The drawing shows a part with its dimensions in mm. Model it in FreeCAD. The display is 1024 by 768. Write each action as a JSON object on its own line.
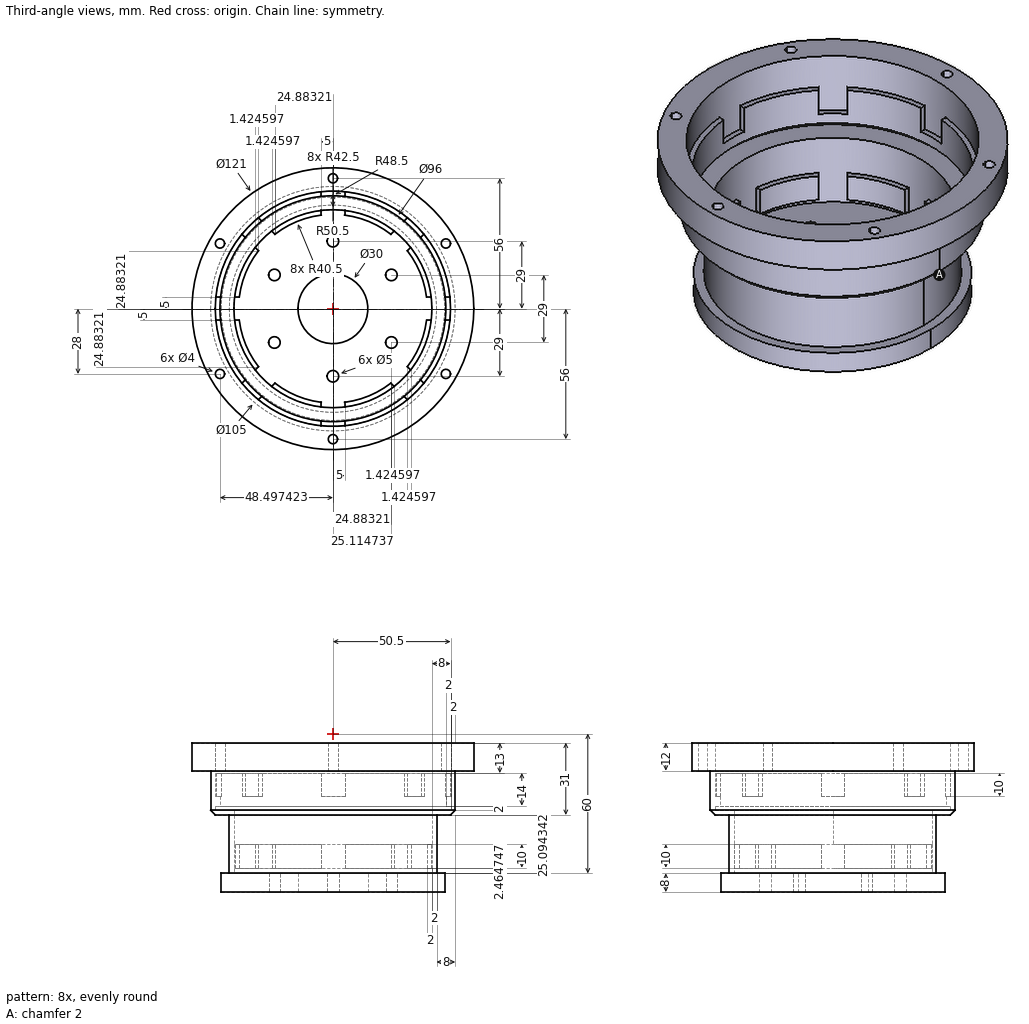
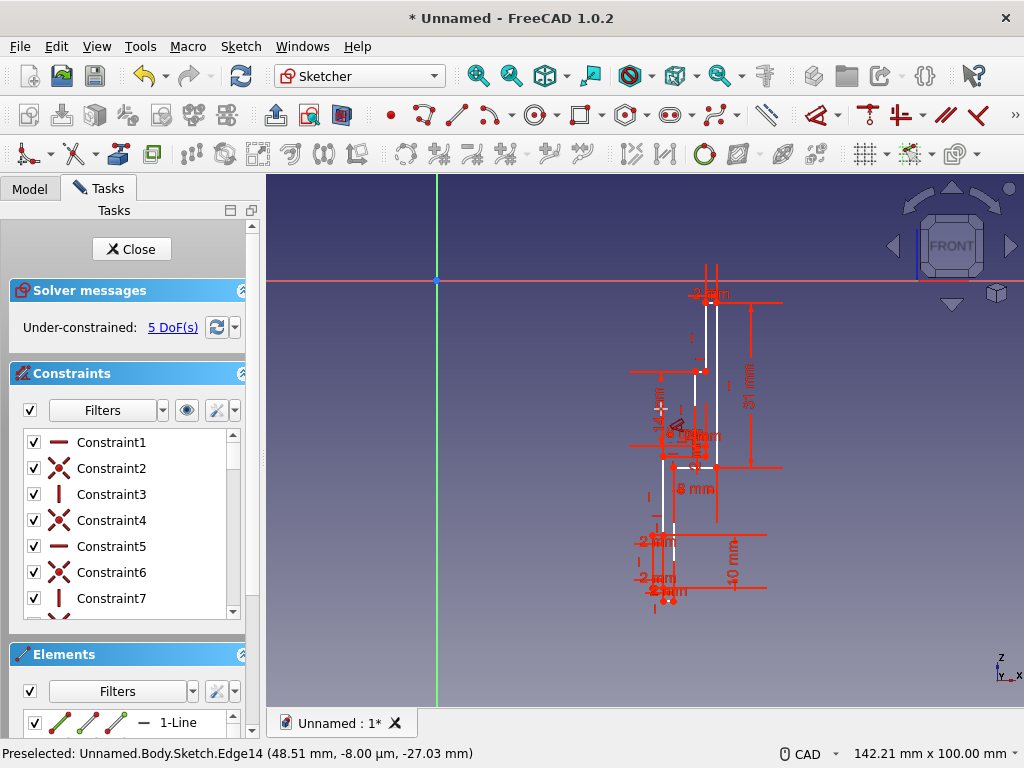
{"action": "scroll", "coordinate": [706, 351], "scroll_direction": "up", "scroll_amount": 2}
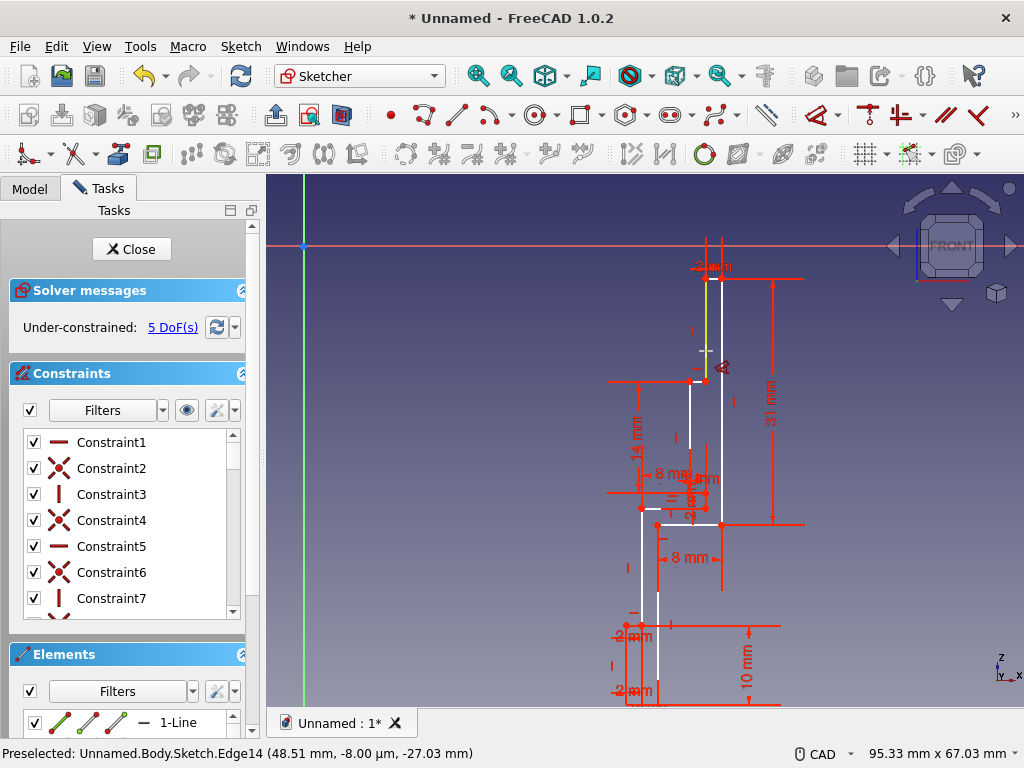
{"action": "left_click", "coordinate": [706, 351]}
{"action": "left_click", "coordinate": [740, 330]}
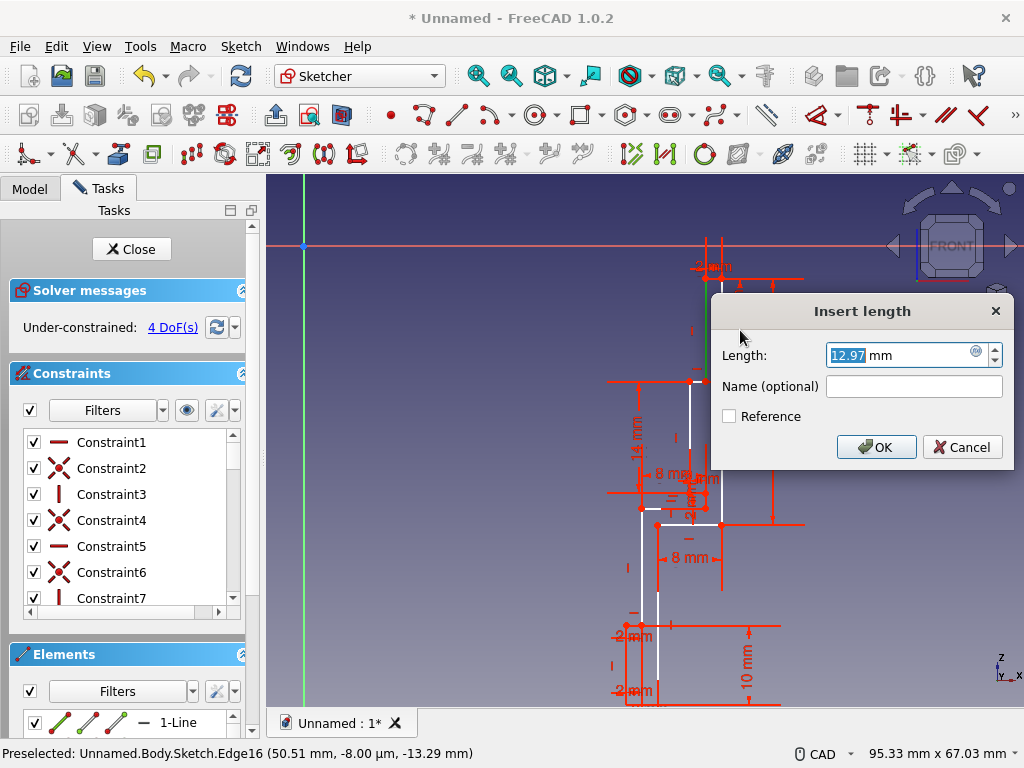
{"action": "type", "text": "13"}
{"action": "key", "text": "Return"}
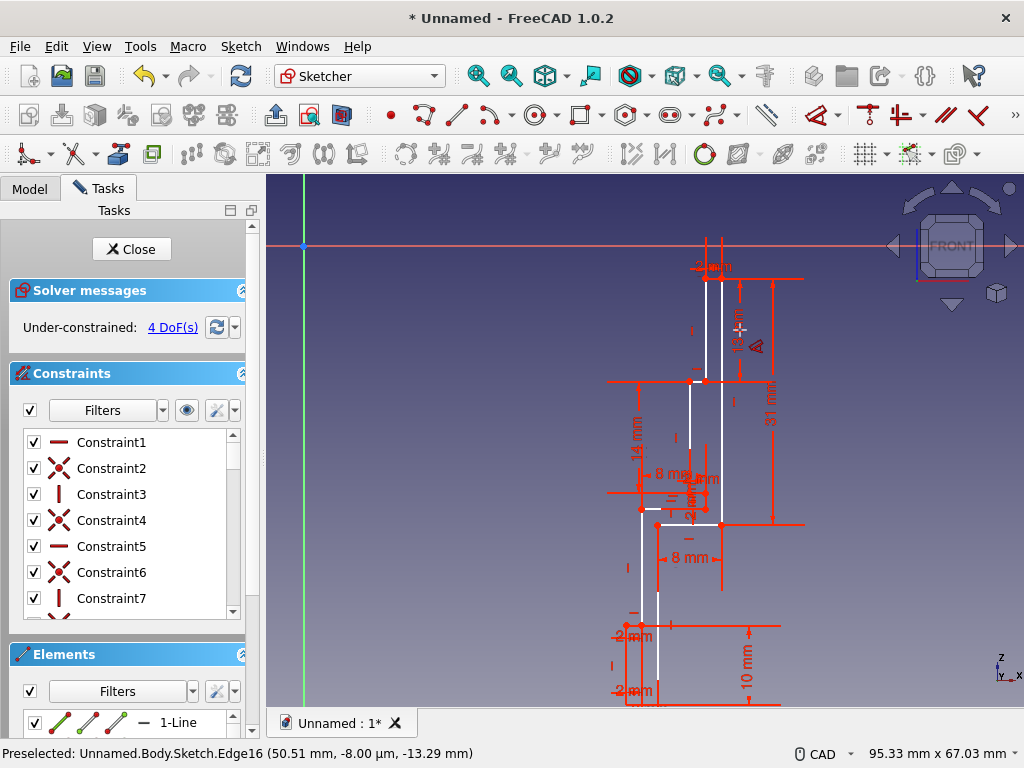
{"action": "scroll", "coordinate": [706, 350], "scroll_direction": "down", "scroll_amount": 2}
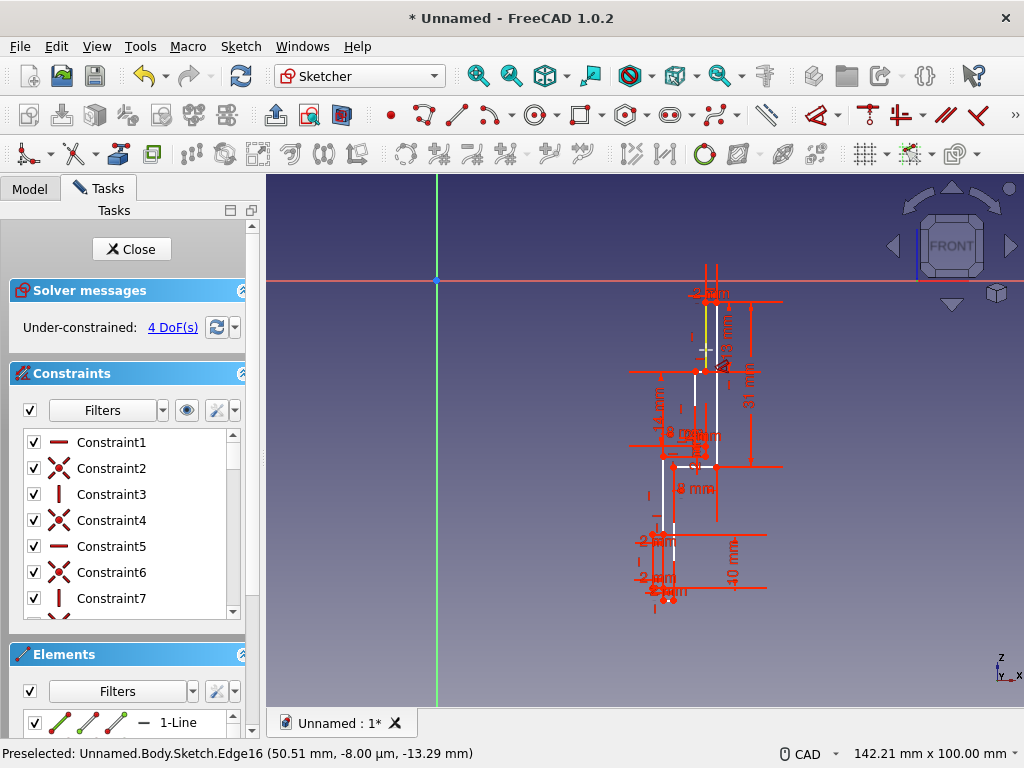
{"action": "left_click", "coordinate": [674, 601]}
{"action": "left_click", "coordinate": [403, 441]}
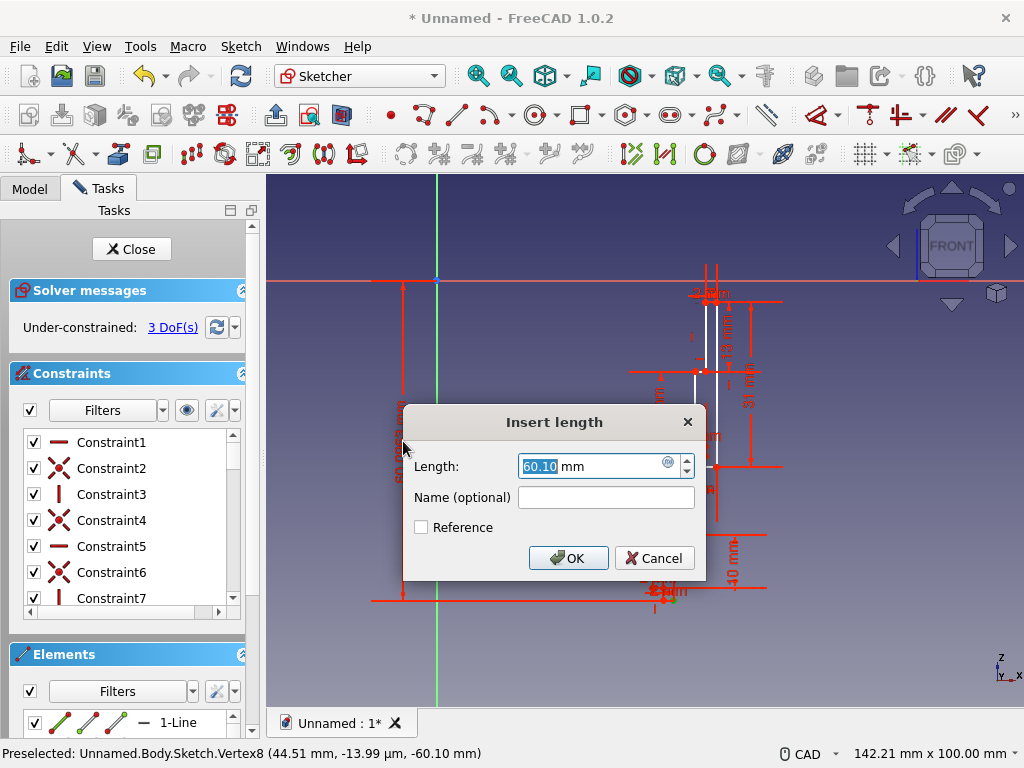
{"action": "type", "text": "60"}
{"action": "key", "text": "Return"}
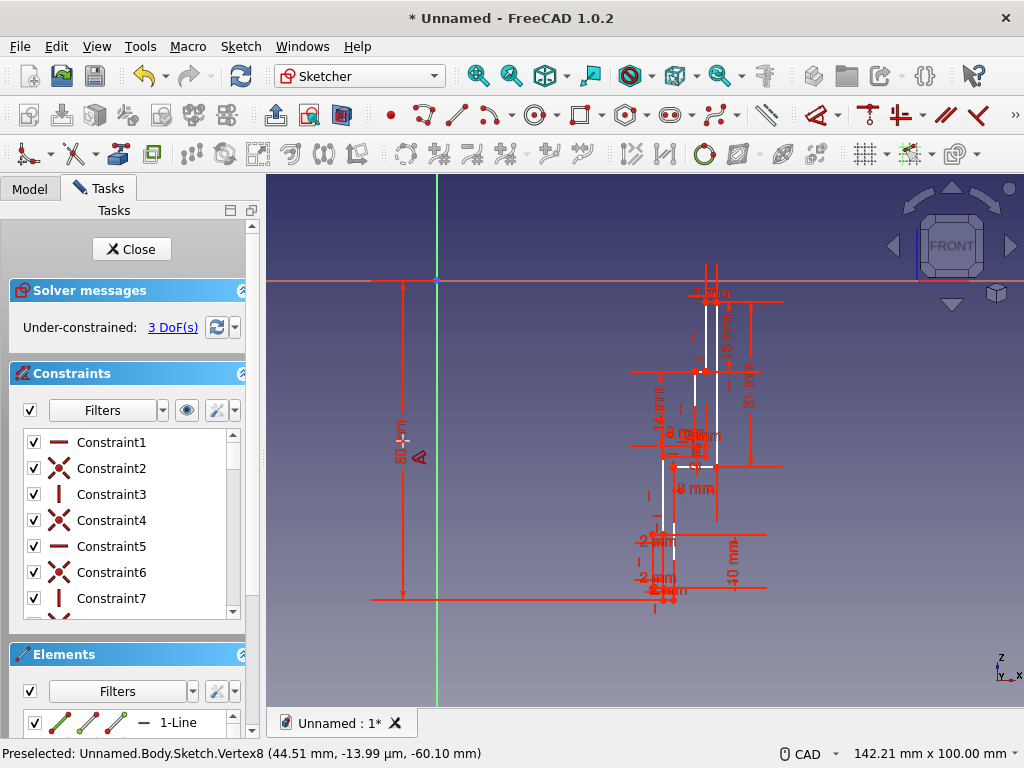
{"action": "left_click", "coordinate": [706, 302]}
{"action": "left_click", "coordinate": [571, 247]}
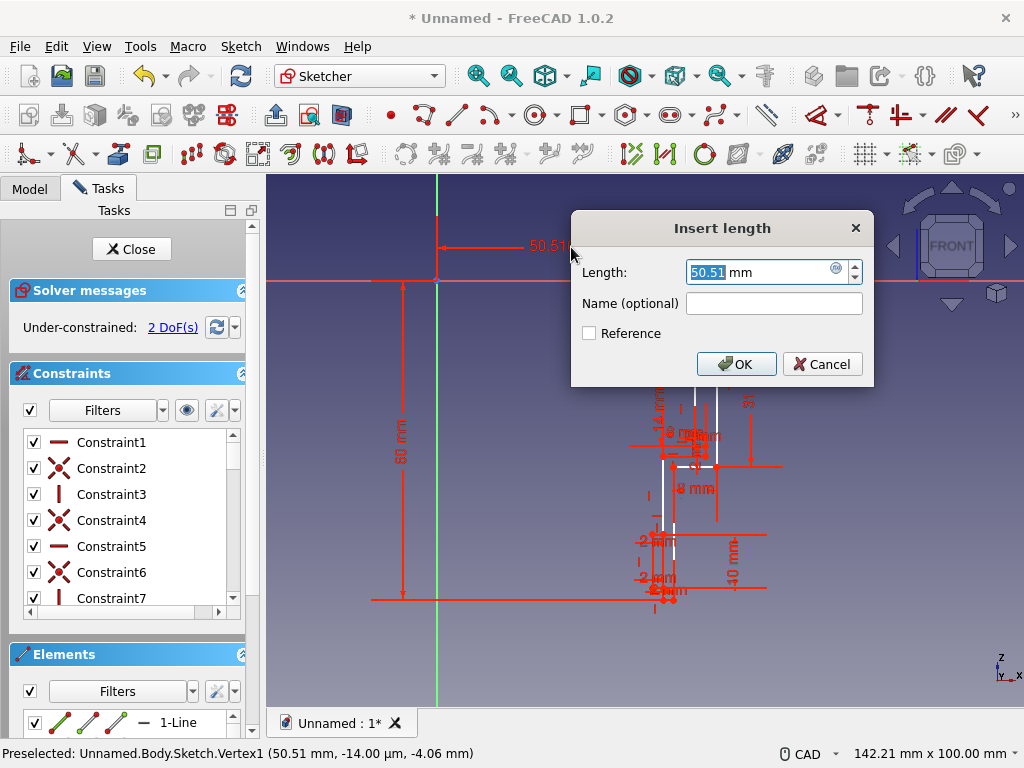
{"action": "type", "text": "50.5"}
{"action": "key", "text": "Return"}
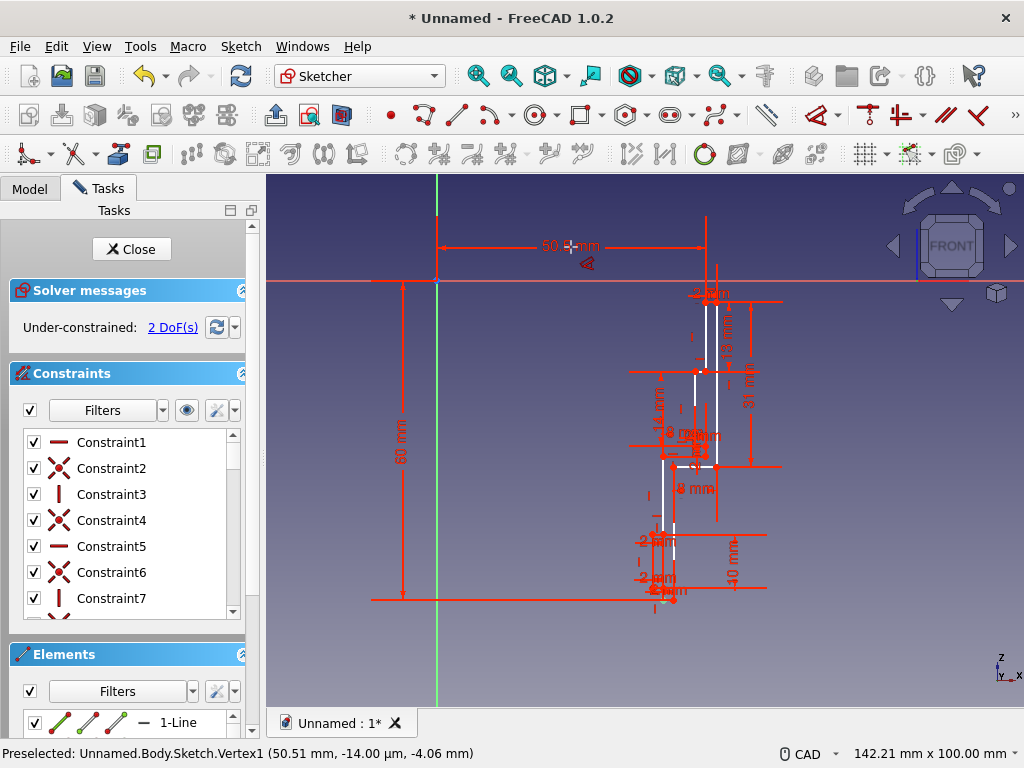
{"action": "scroll", "coordinate": [663, 594], "scroll_direction": "up", "scroll_amount": 6}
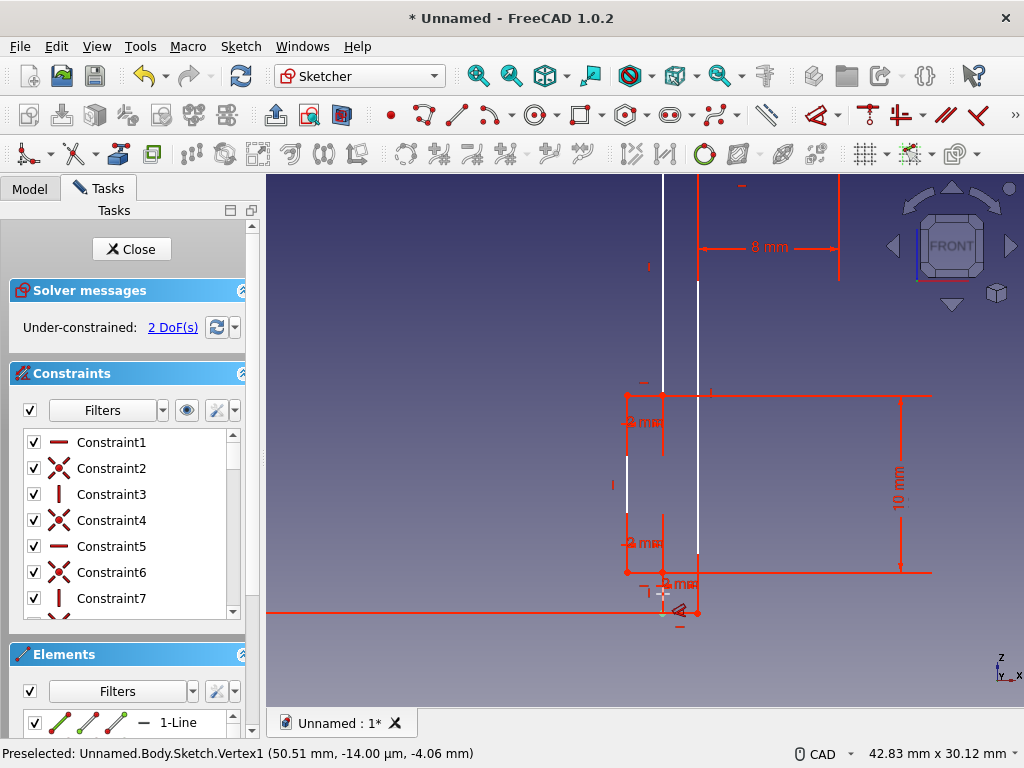
{"action": "left_click", "coordinate": [663, 593]}
{"action": "left_click", "coordinate": [629, 607]}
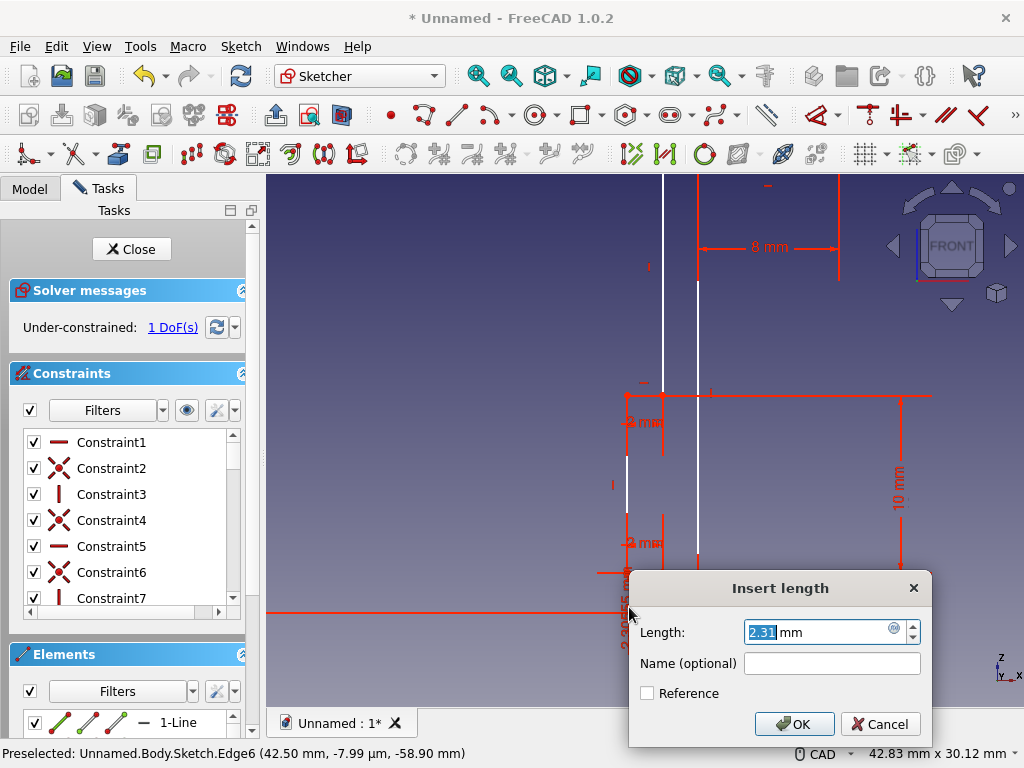
{"action": "type", "text": "2.464747"}
{"action": "key", "text": "Return"}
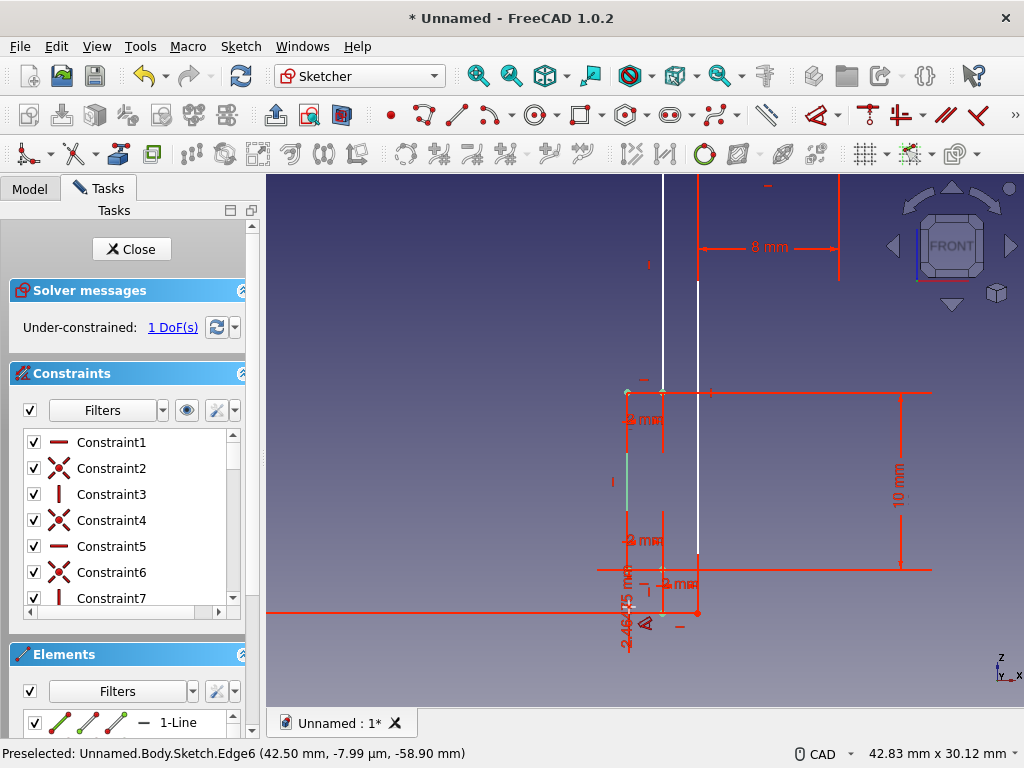
{"action": "left_click", "coordinate": [698, 304]}
{"action": "left_click", "coordinate": [732, 408]}